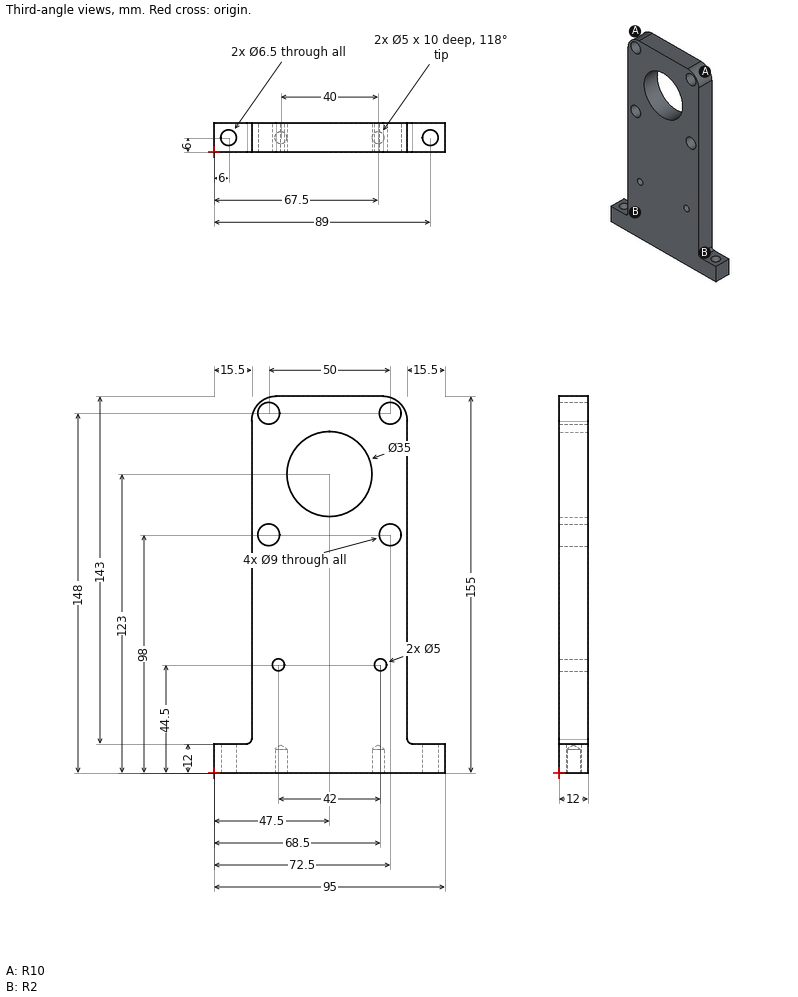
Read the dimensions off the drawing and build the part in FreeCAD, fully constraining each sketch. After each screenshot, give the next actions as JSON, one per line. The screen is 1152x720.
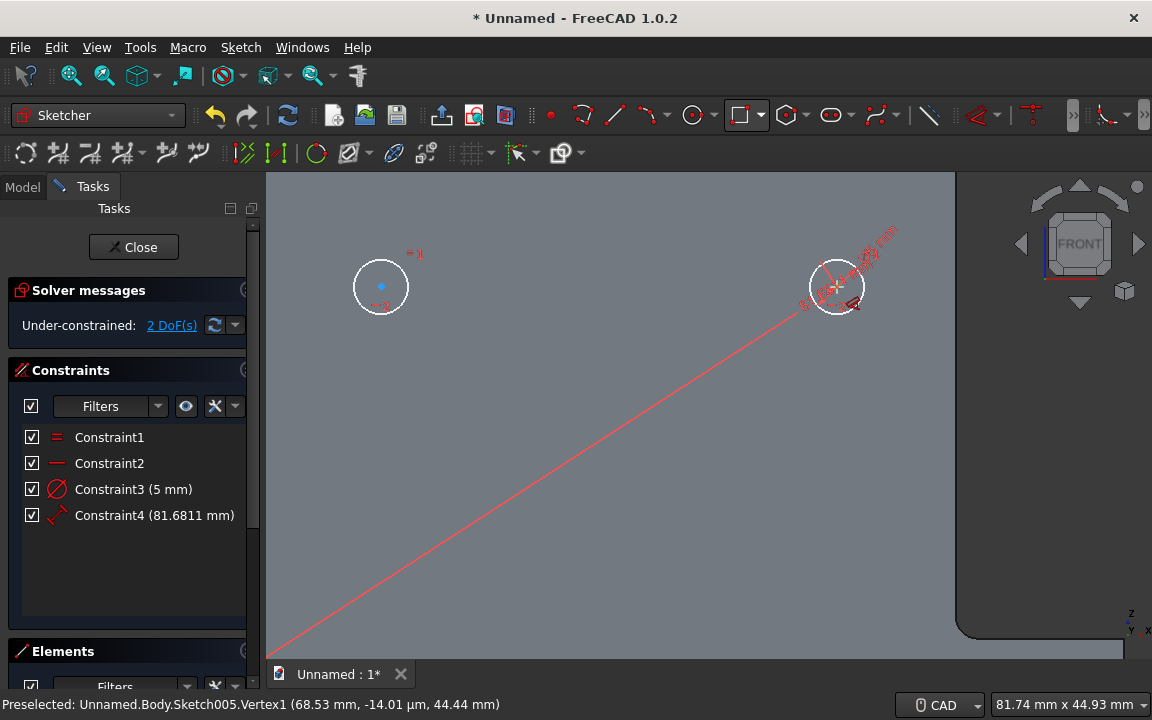
{"action": "left_click", "coordinate": [381, 287]}
{"action": "left_click", "coordinate": [609, 253]}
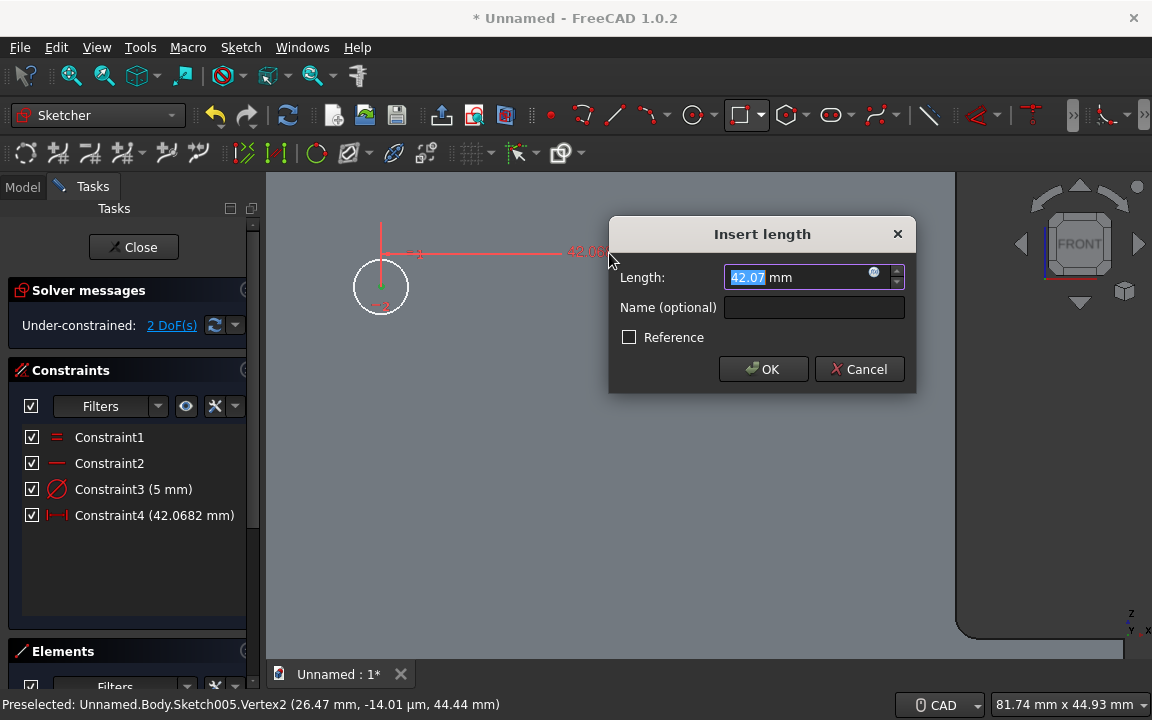
{"action": "type", "text": "42"}
{"action": "key", "text": "Return"}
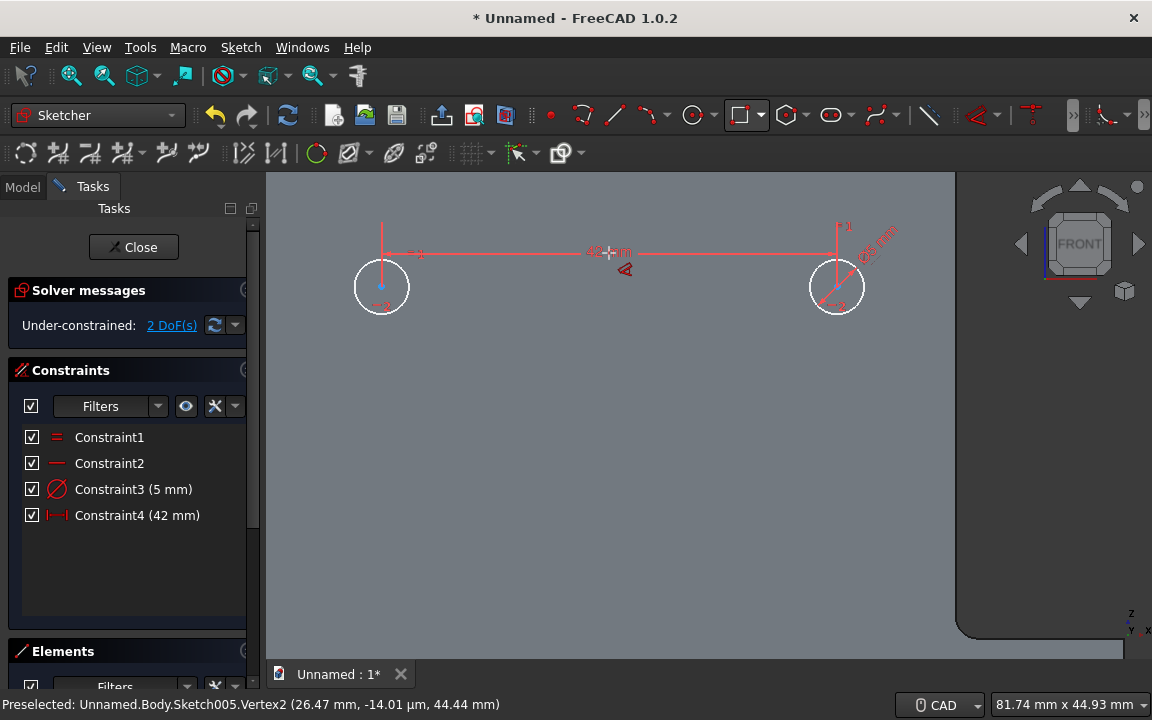
{"action": "left_click", "coordinate": [837, 287]}
{"action": "left_click", "coordinate": [441, 253]}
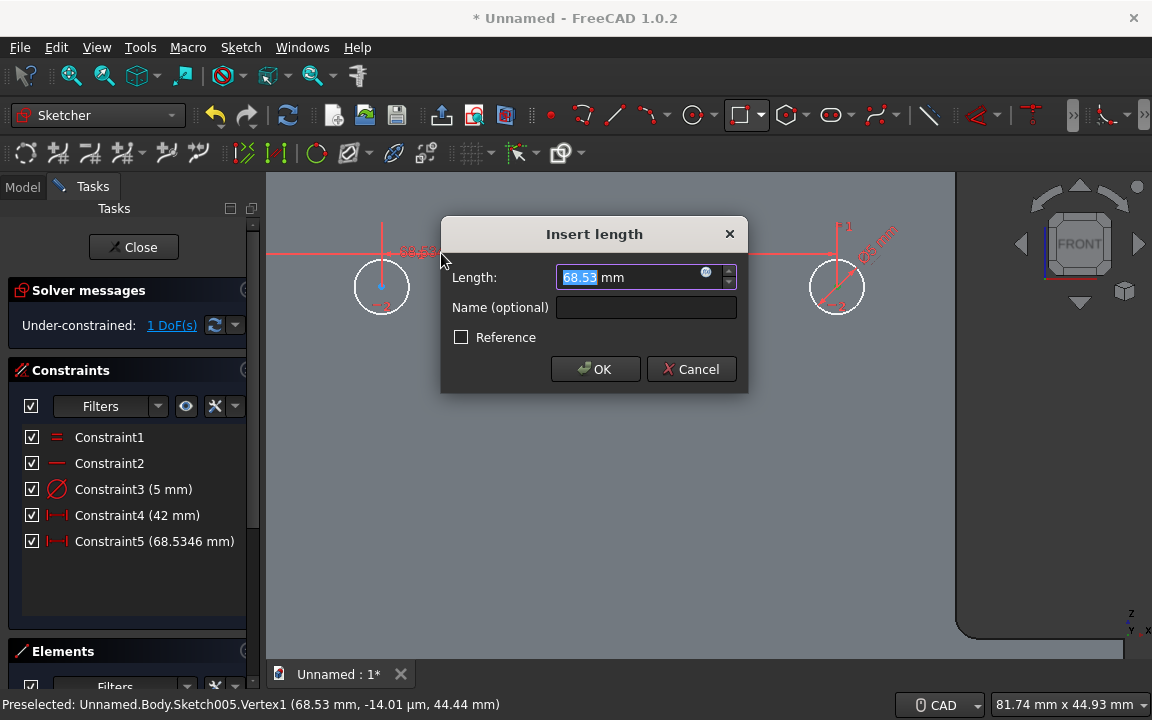
{"action": "type", "text": "68.5"}
{"action": "key", "text": "Return"}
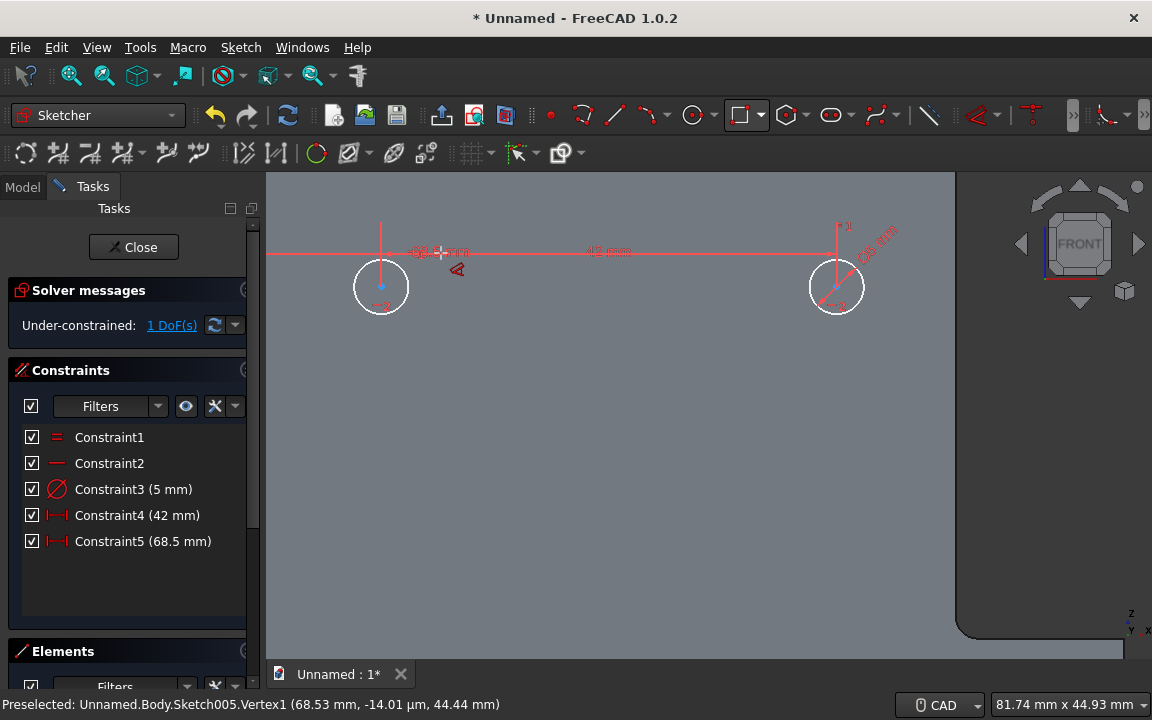
{"action": "left_click", "coordinate": [837, 287]}
{"action": "left_click", "coordinate": [871, 459]}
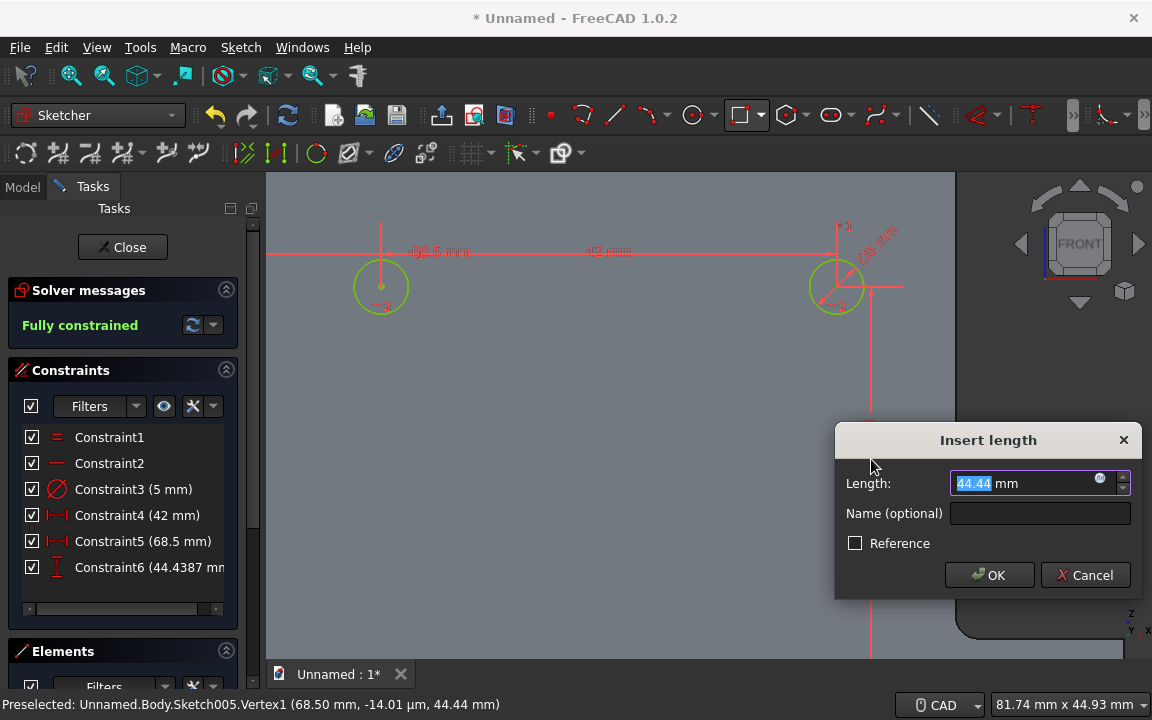
{"action": "type", "text": "44.5"}
{"action": "key", "text": "Return"}
{"action": "key", "text": "Escape"}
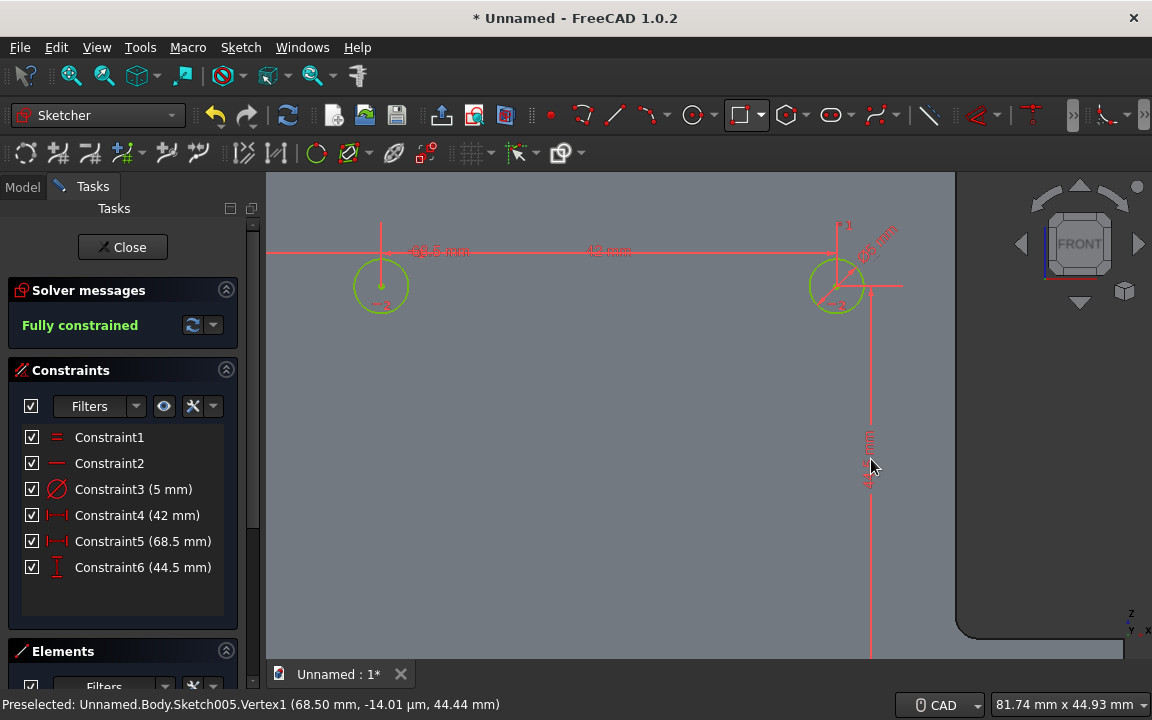
{"action": "left_click", "coordinate": [123, 247]}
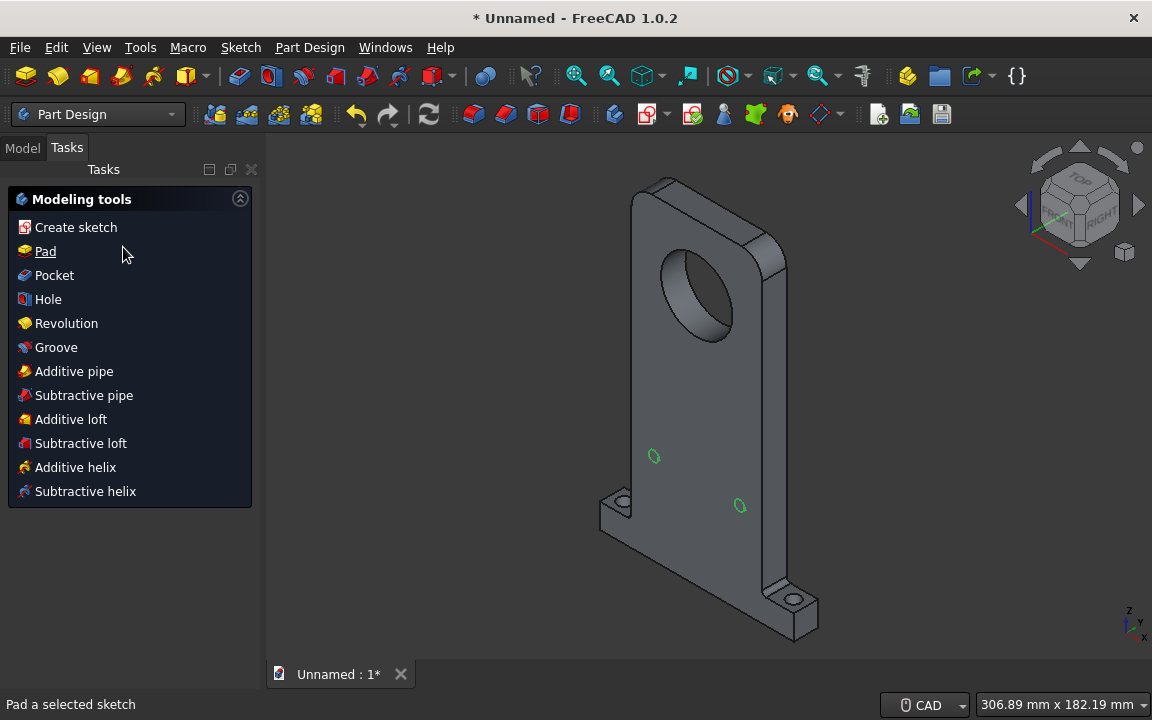
{"action": "left_click", "coordinate": [240, 76]}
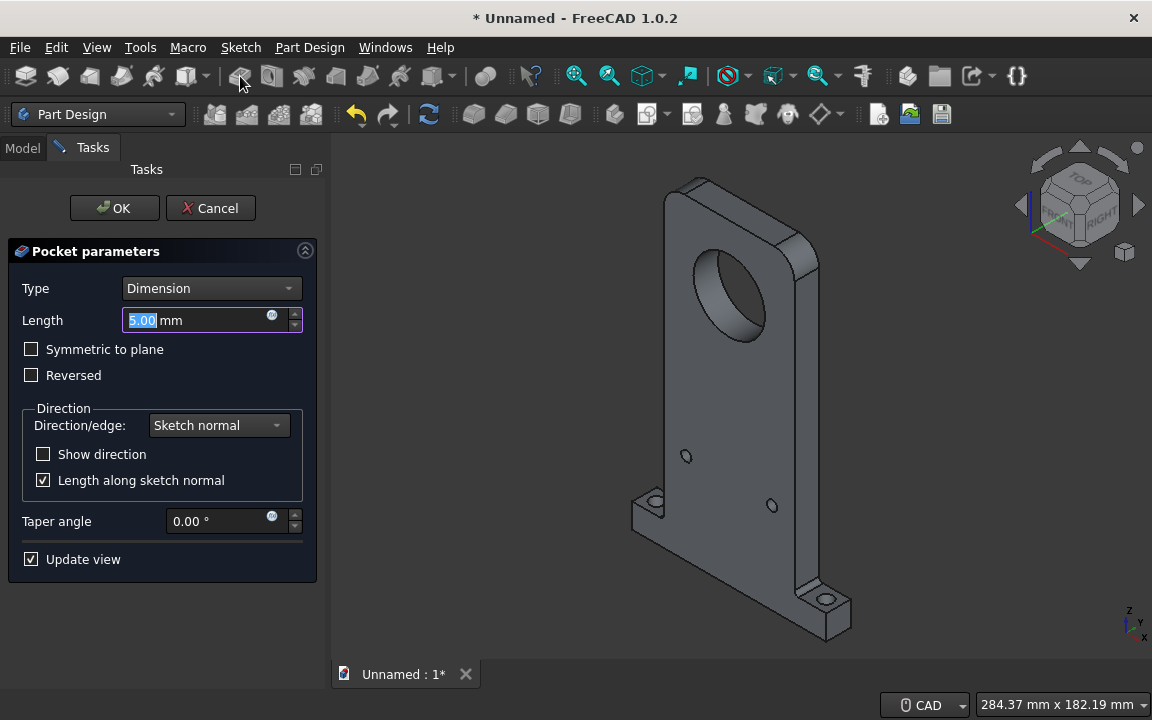
{"action": "left_click", "coordinate": [212, 288]}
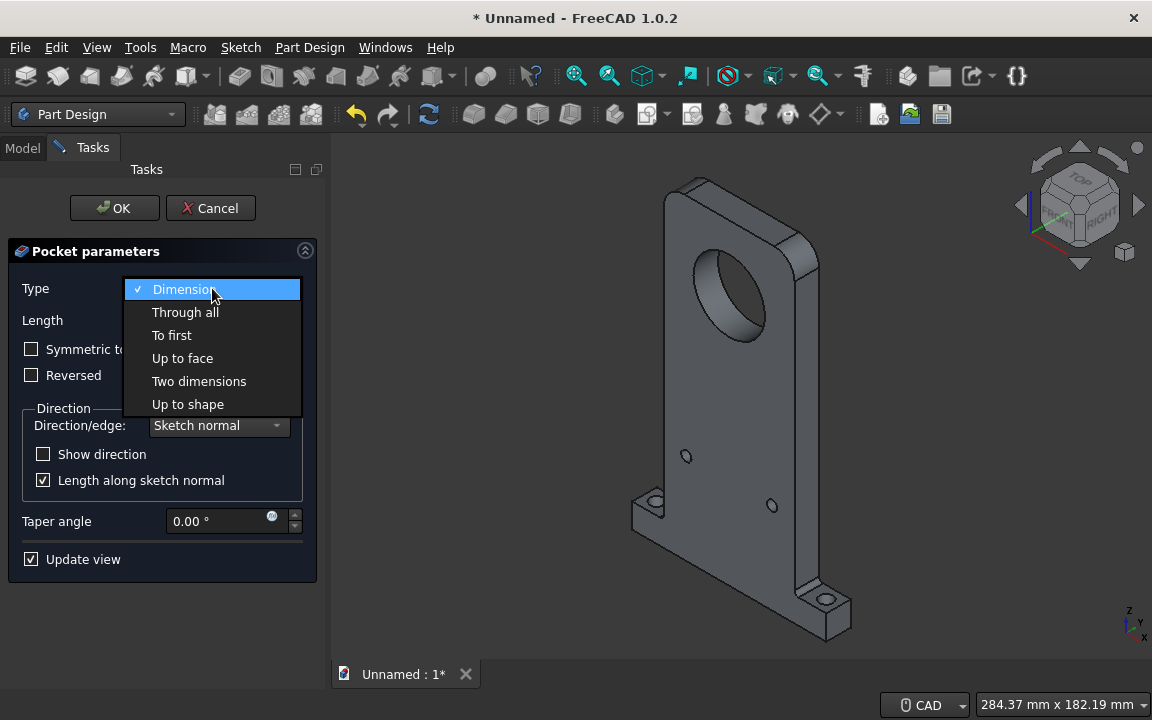
{"action": "left_click", "coordinate": [212, 312]}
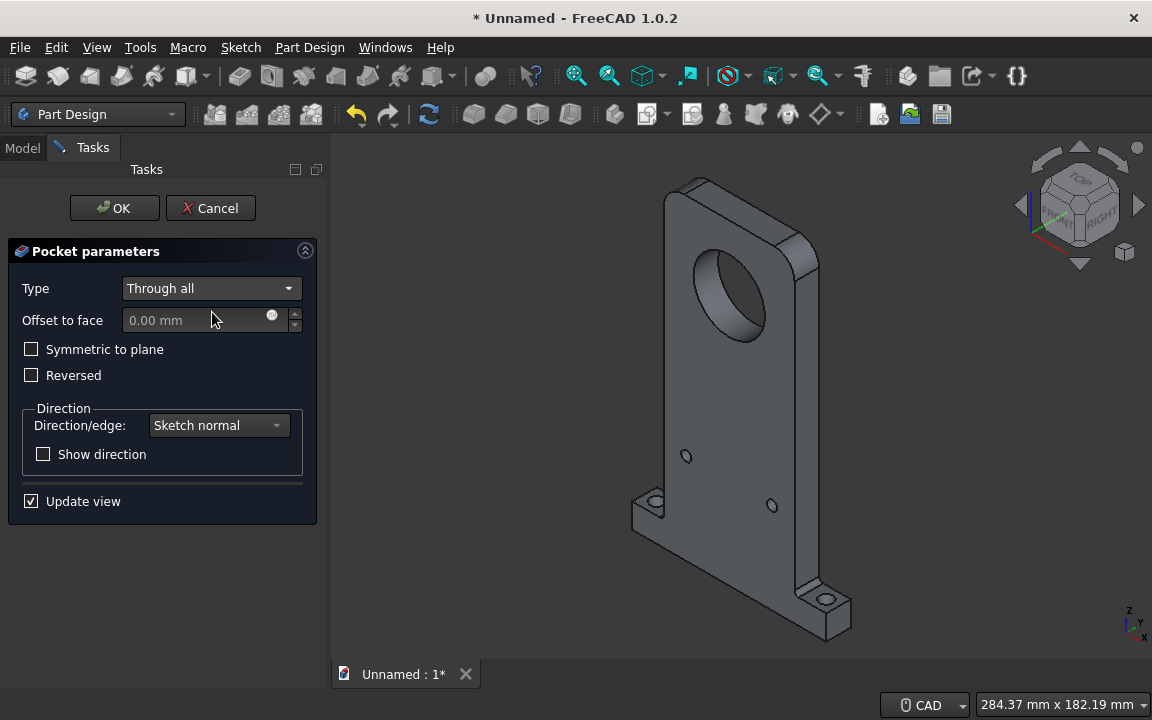
{"action": "left_click", "coordinate": [115, 208]}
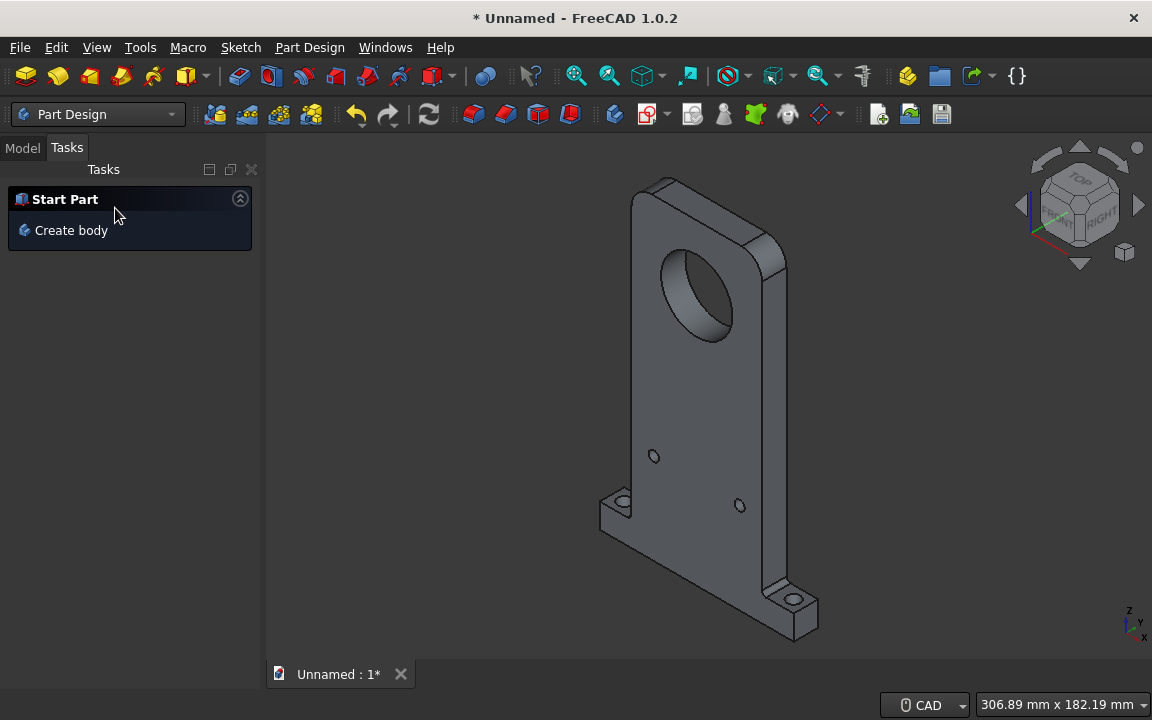
{"action": "left_click", "coordinate": [697, 402]}